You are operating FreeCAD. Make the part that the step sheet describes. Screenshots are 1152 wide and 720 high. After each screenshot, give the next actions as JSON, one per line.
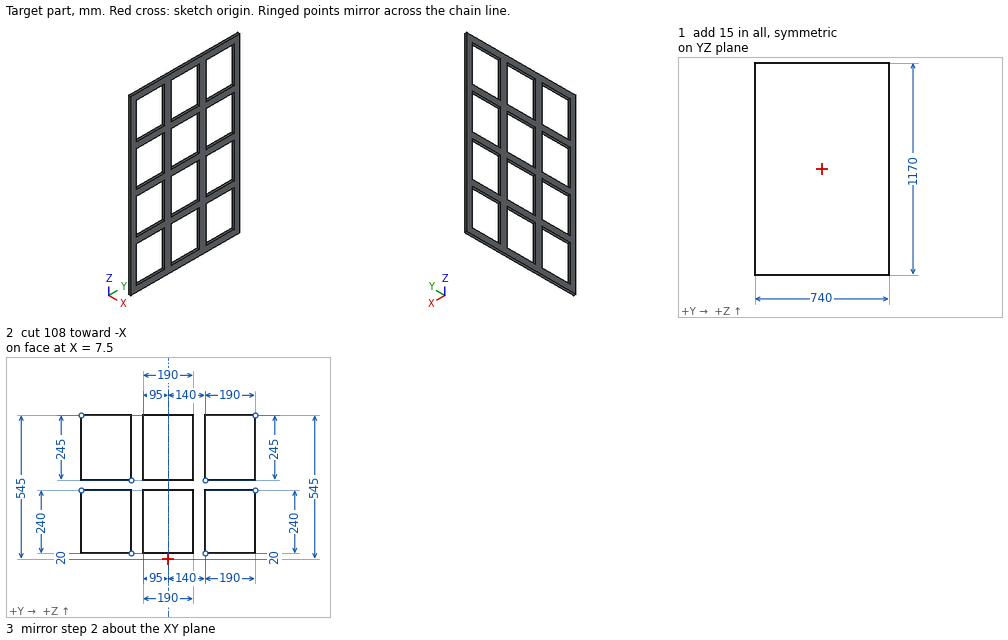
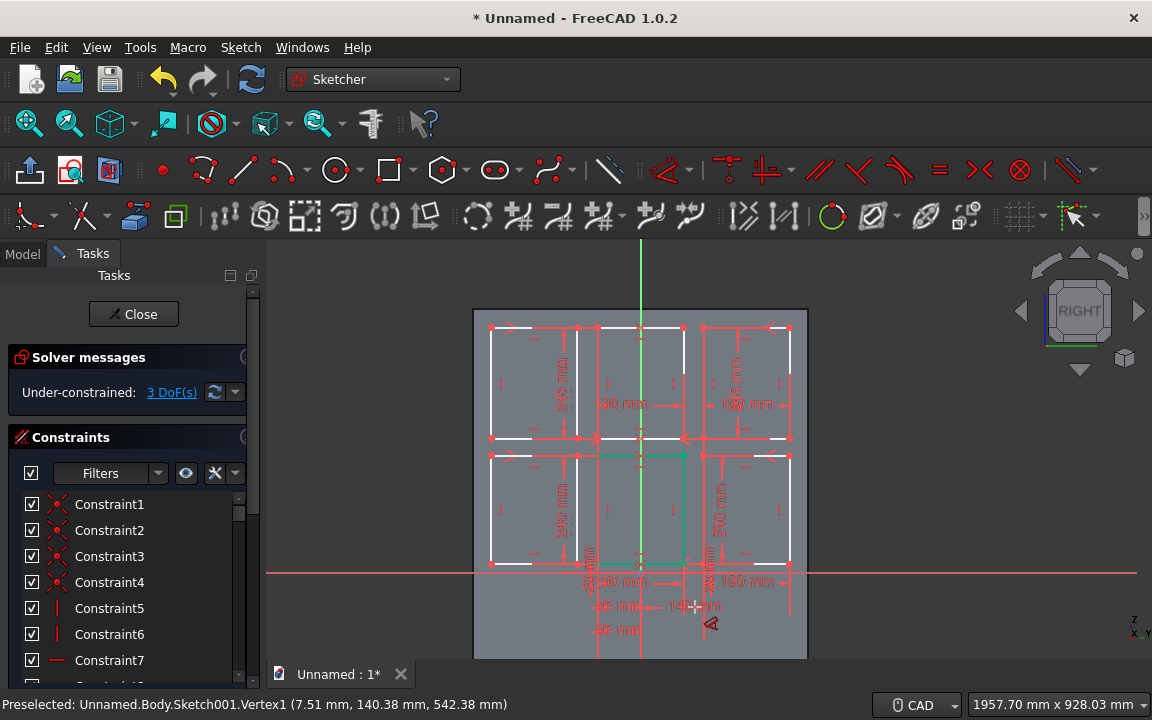
{"action": "left_click", "coordinate": [704, 328]}
{"action": "left_click", "coordinate": [738, 536]}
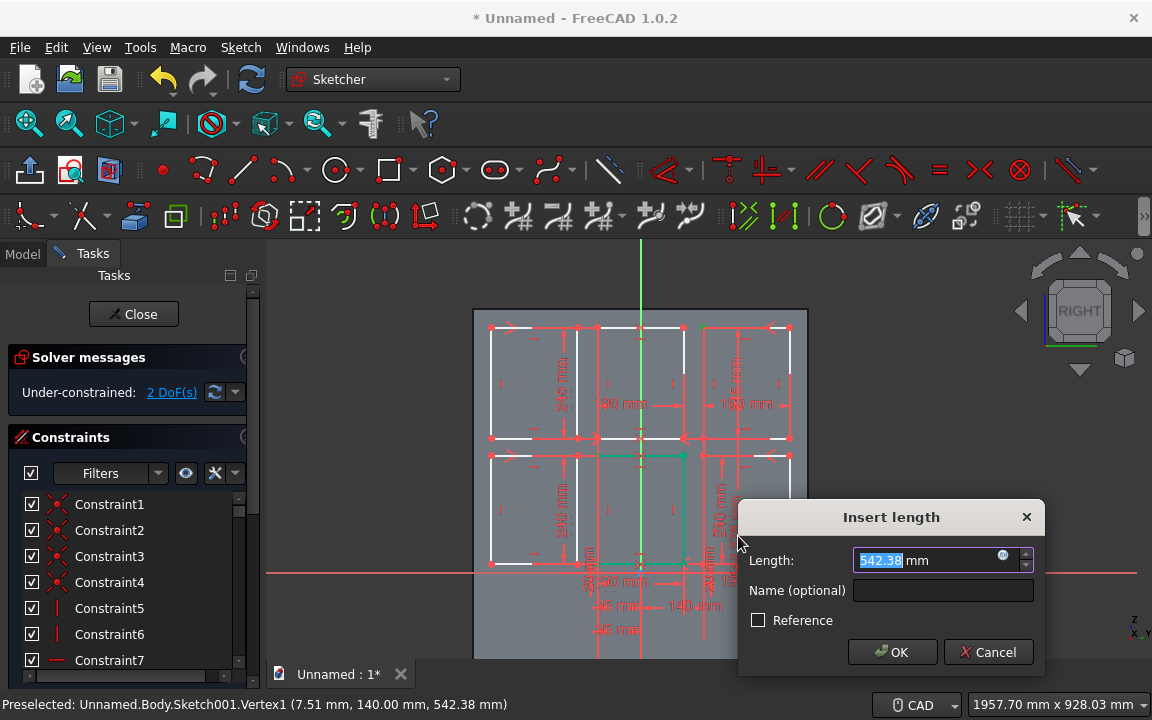
{"action": "type", "text": "545"}
{"action": "key", "text": "Return"}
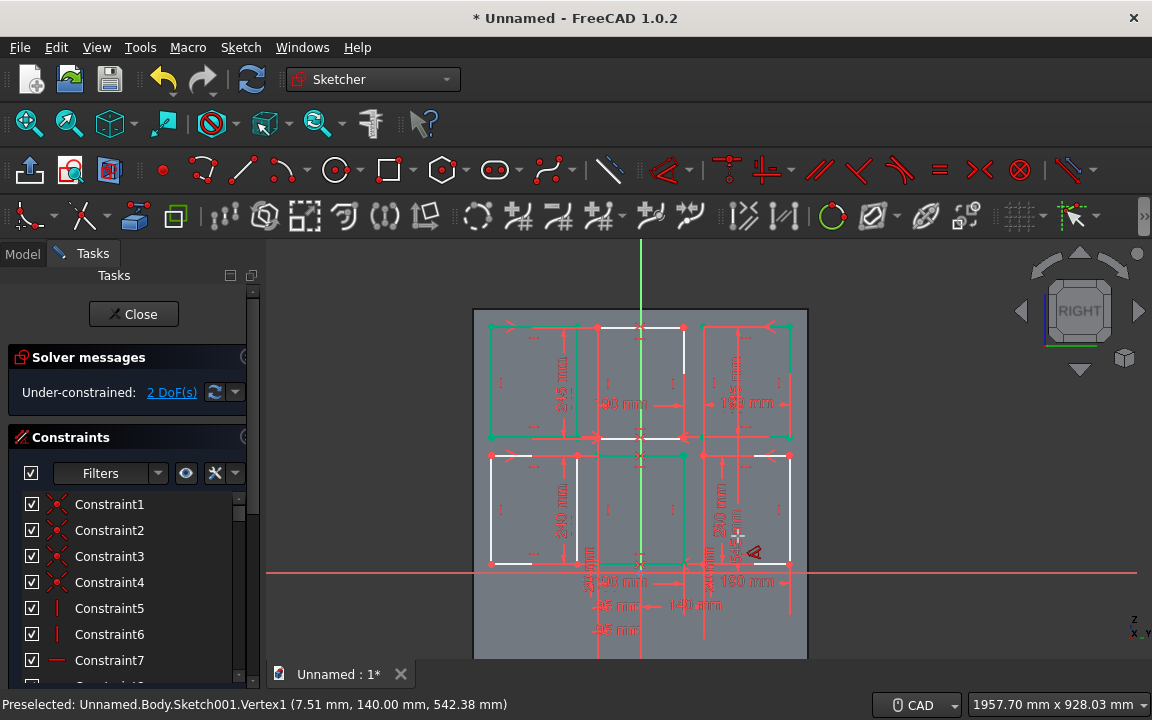
{"action": "left_click", "coordinate": [598, 328]}
{"action": "left_click", "coordinate": [564, 536]}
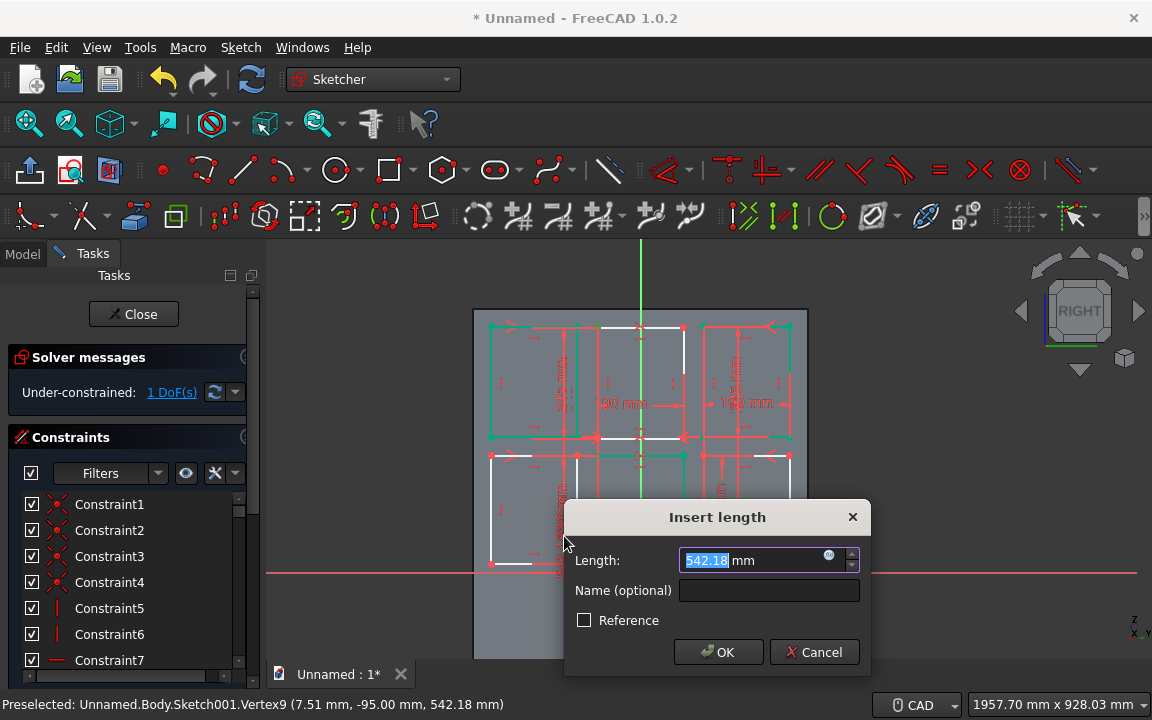
{"action": "type", "text": "545"}
{"action": "key", "text": "Return"}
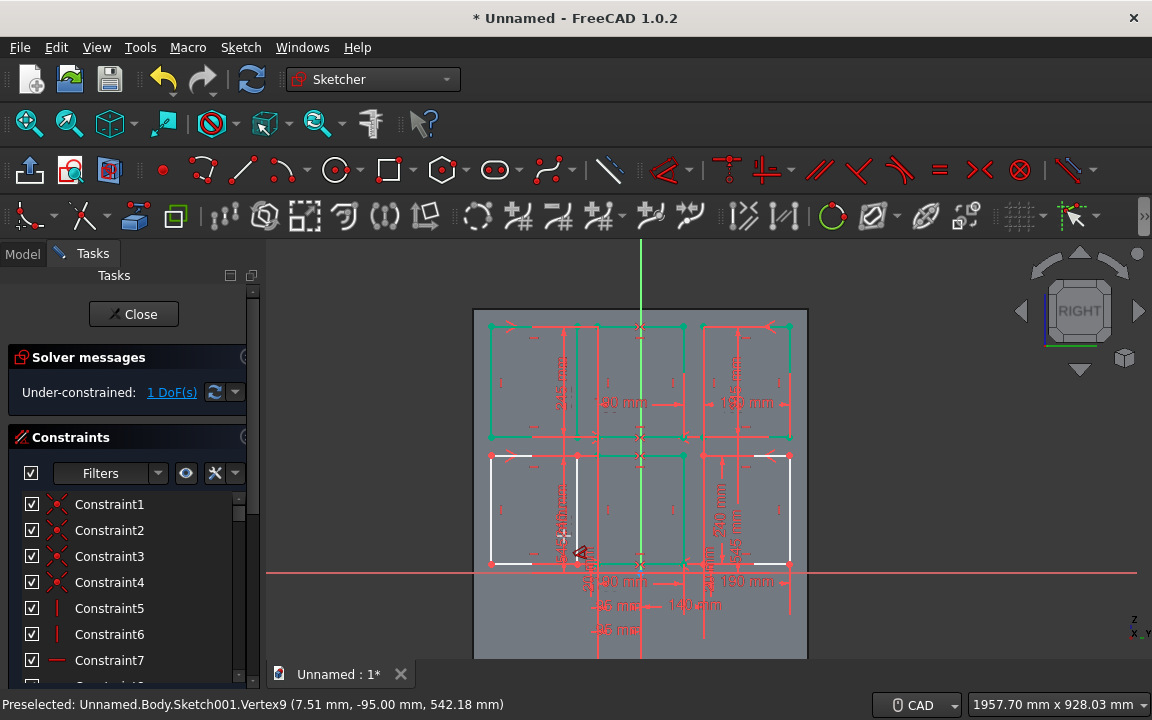
{"action": "left_click", "coordinate": [704, 456]}
{"action": "left_click", "coordinate": [658, 374]}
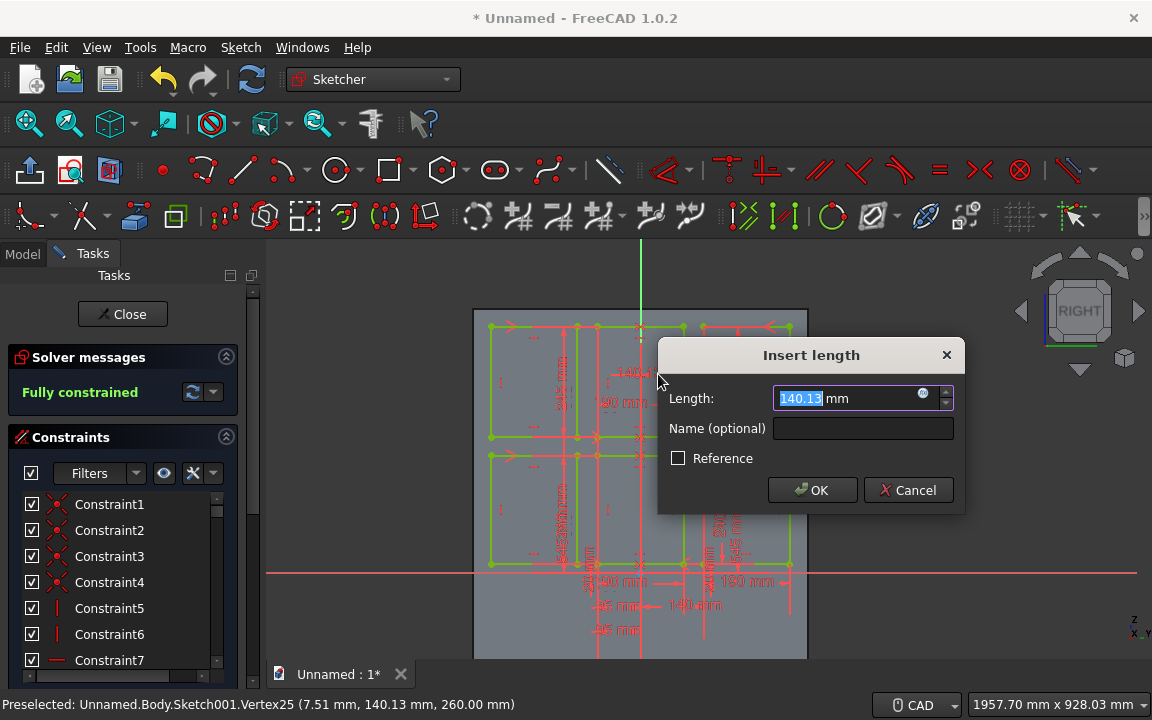
{"action": "type", "text": "140"}
{"action": "key", "text": "Return"}
{"action": "key", "text": "Escape"}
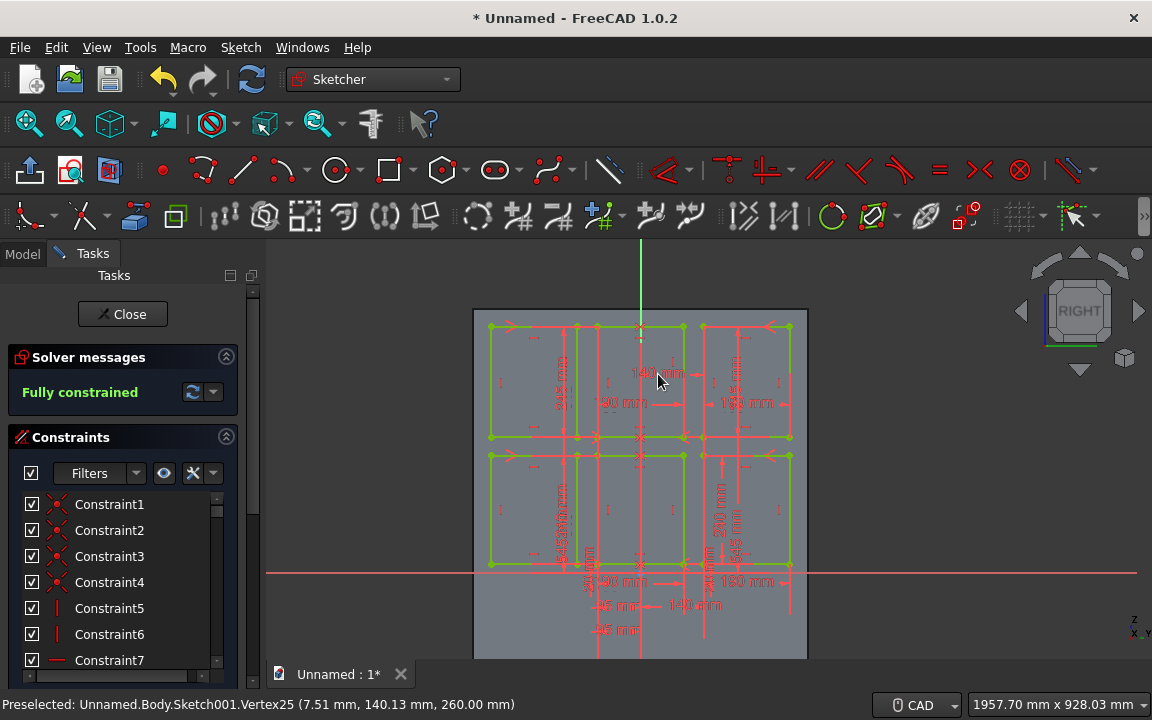
{"action": "left_click", "coordinate": [123, 314]}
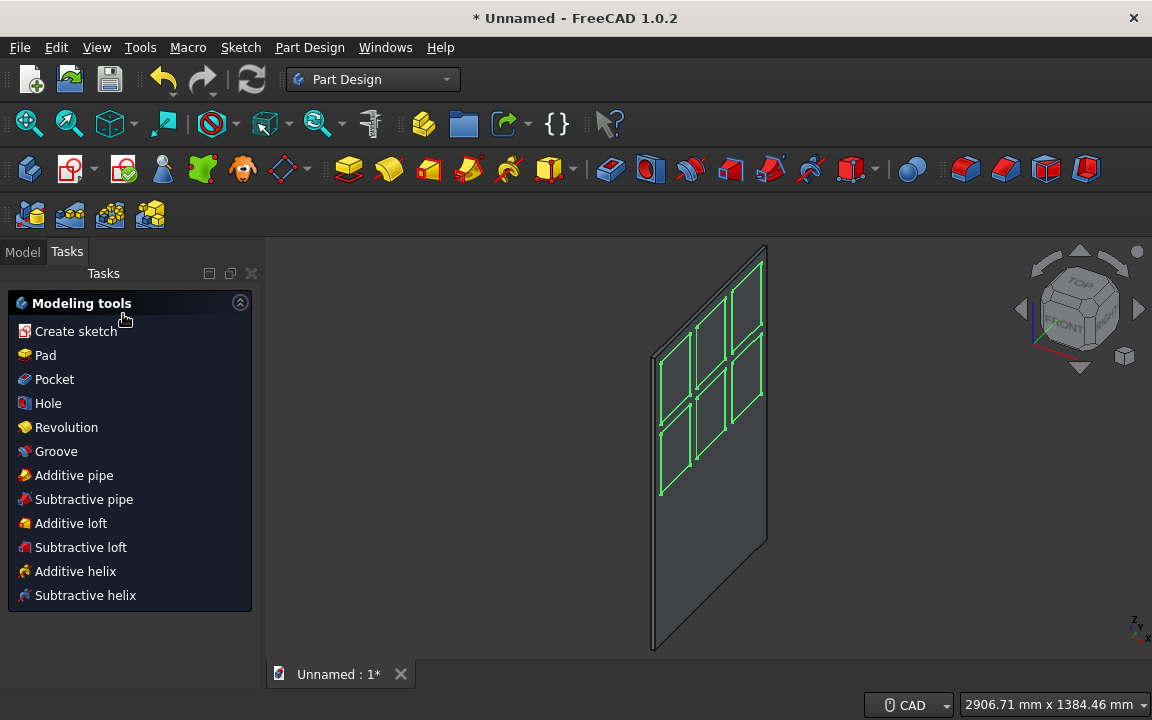
{"action": "left_click", "coordinate": [612, 170]}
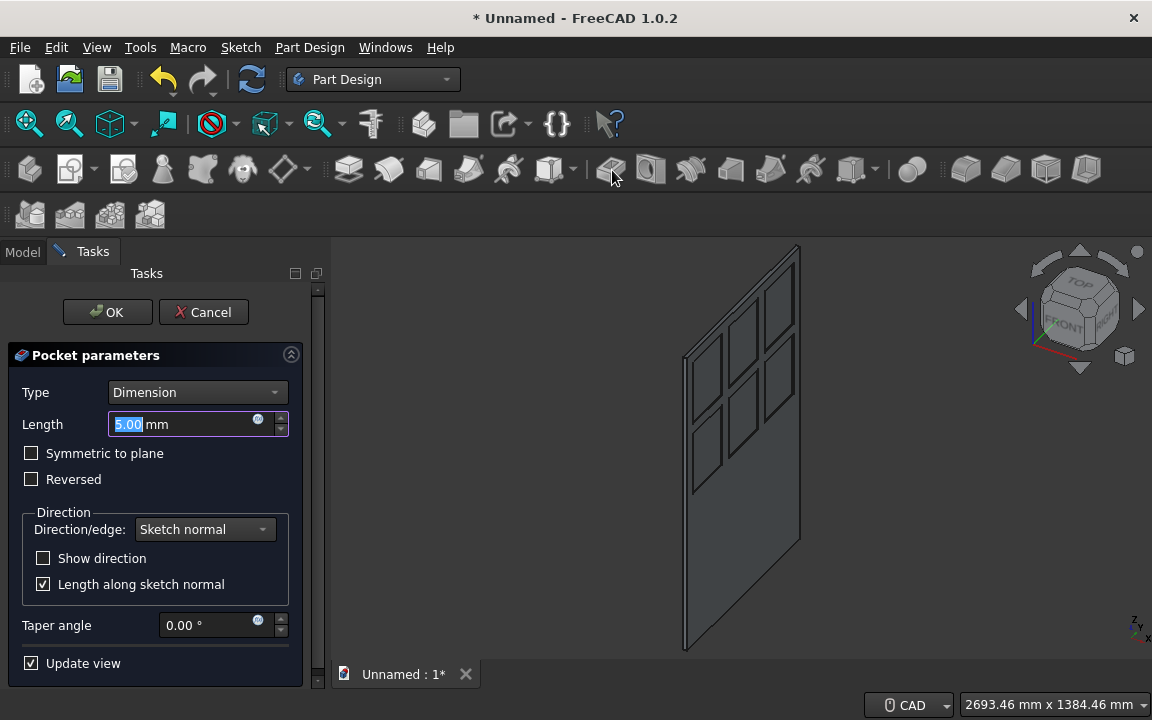
{"action": "type", "text": "108"}
{"action": "key", "text": "Tab"}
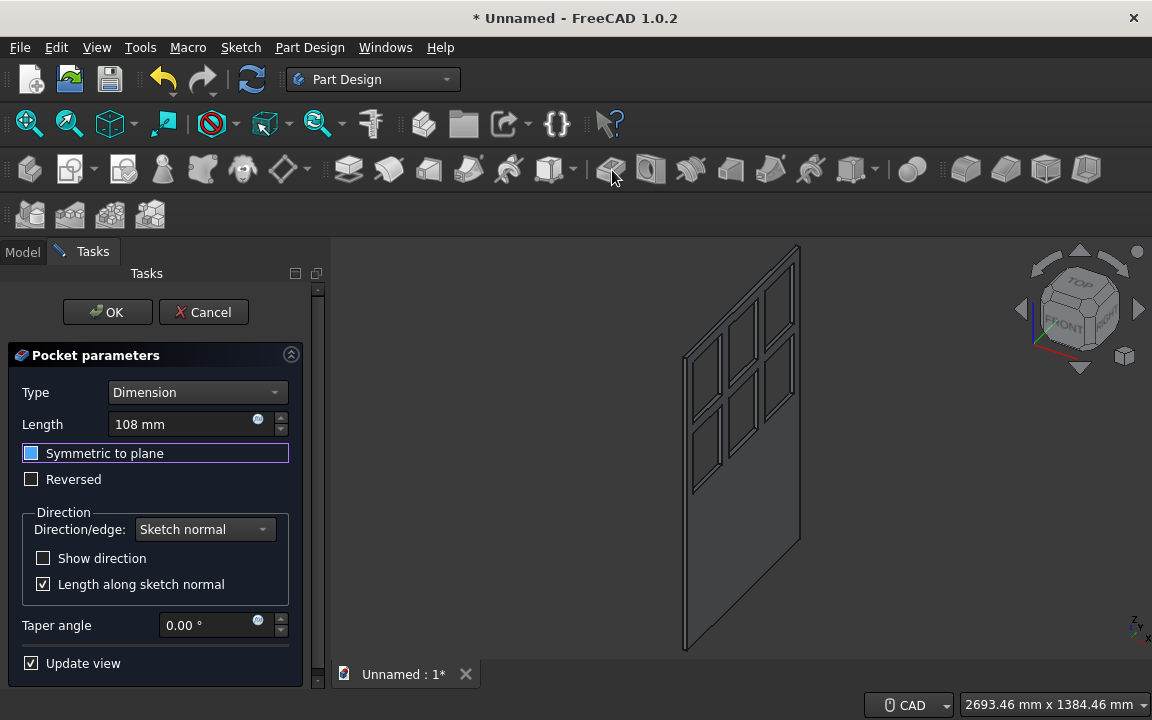
{"action": "left_click", "coordinate": [108, 312]}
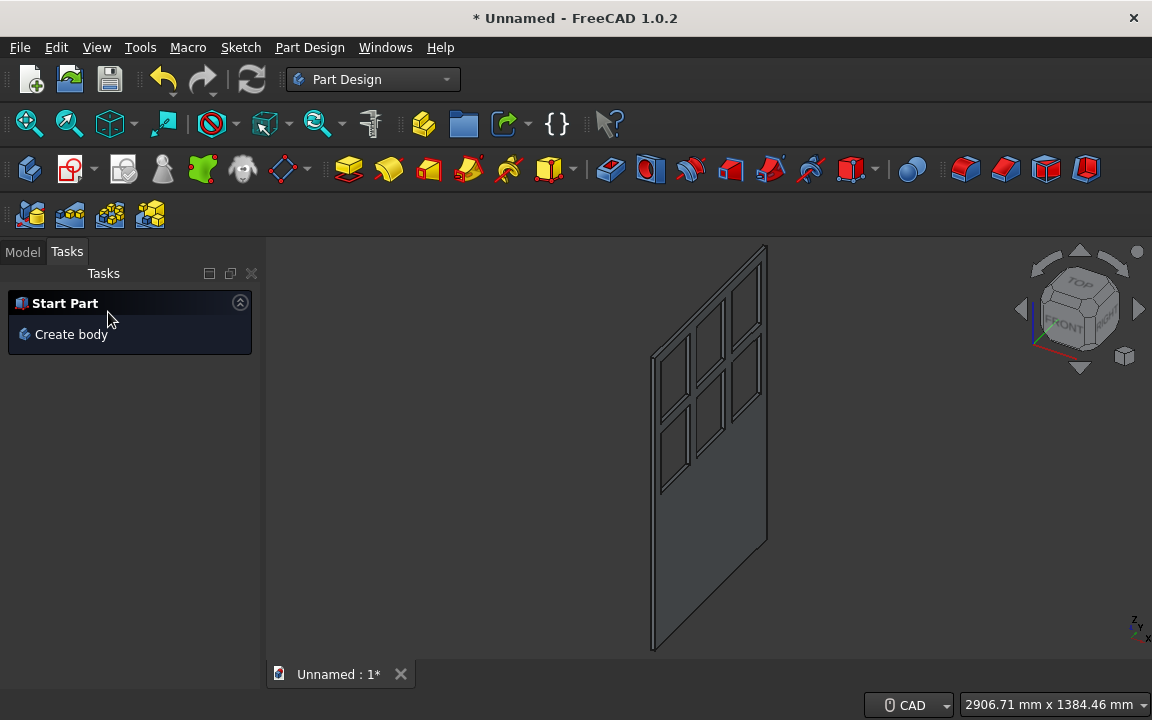
{"action": "left_click", "coordinate": [23, 251]}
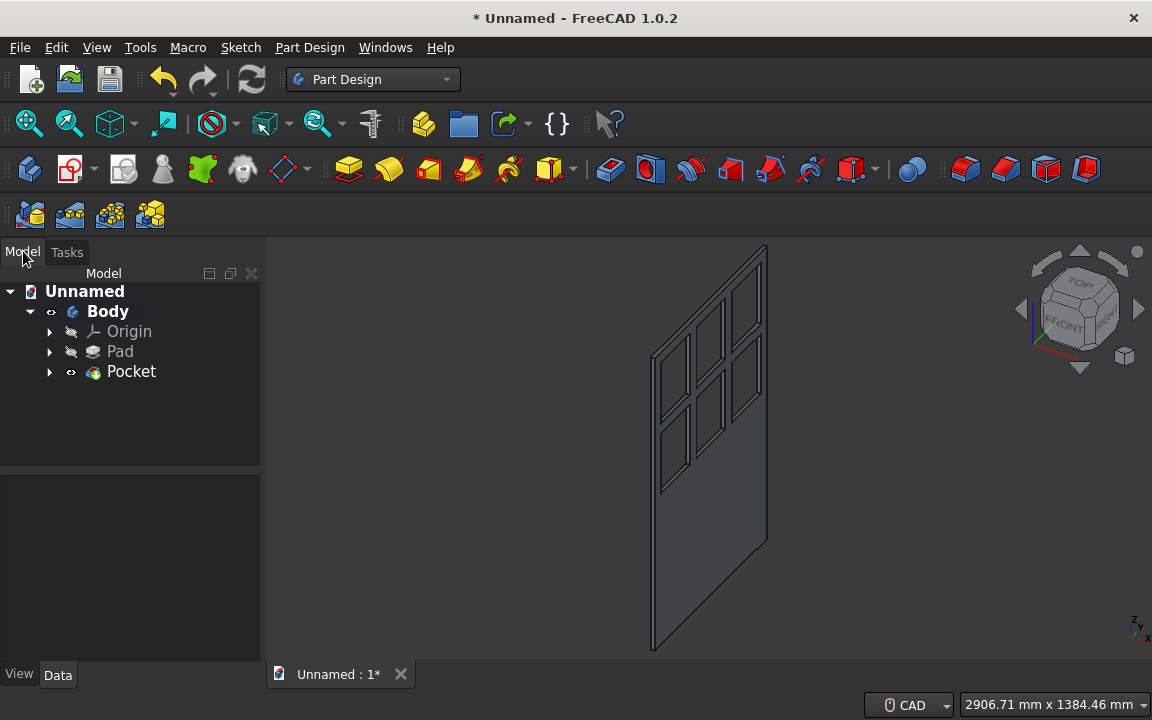
{"action": "left_click", "coordinate": [116, 372]}